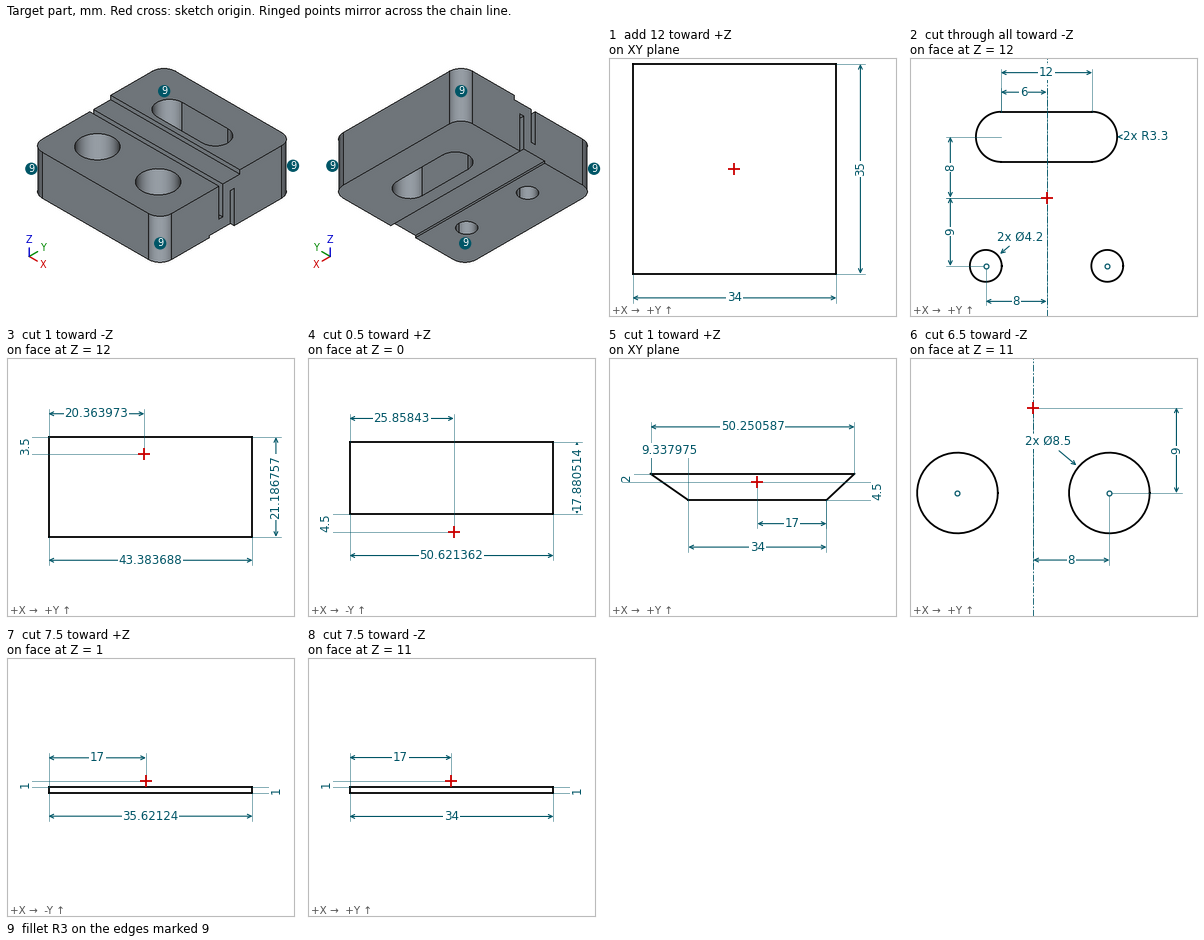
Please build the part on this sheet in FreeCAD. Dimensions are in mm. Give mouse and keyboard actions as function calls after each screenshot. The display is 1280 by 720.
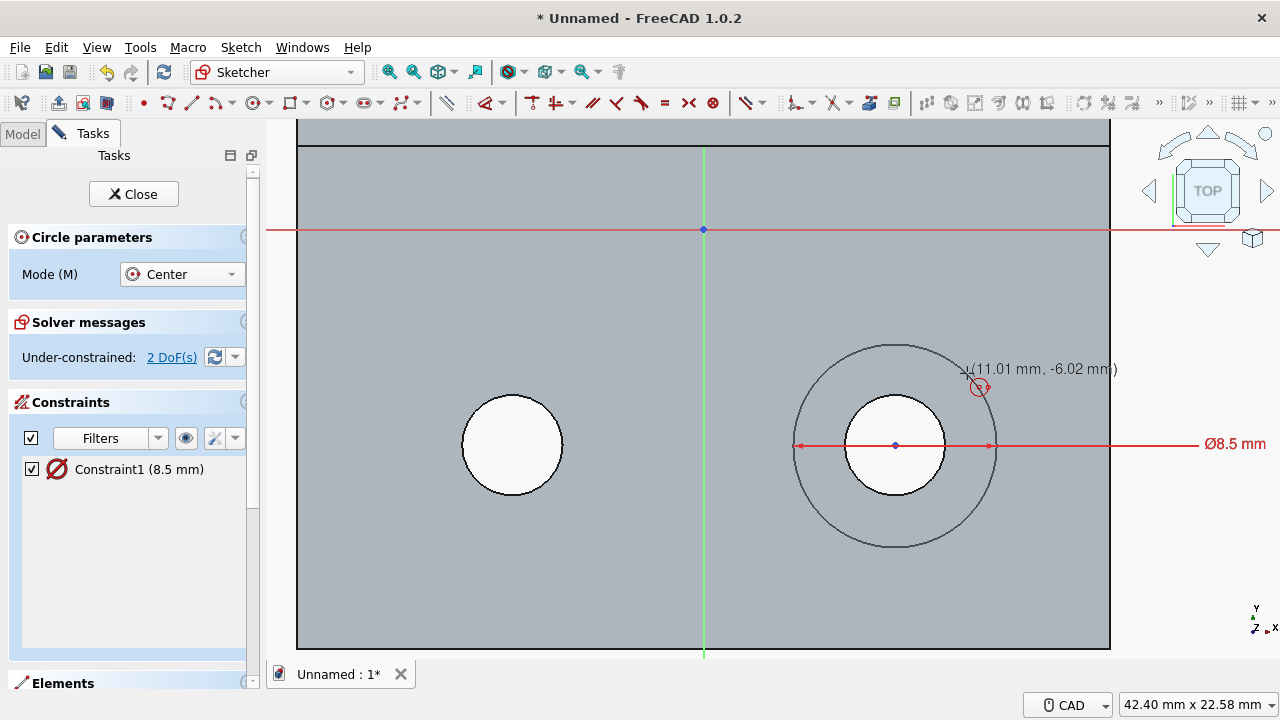
click(512, 445)
move(584, 373)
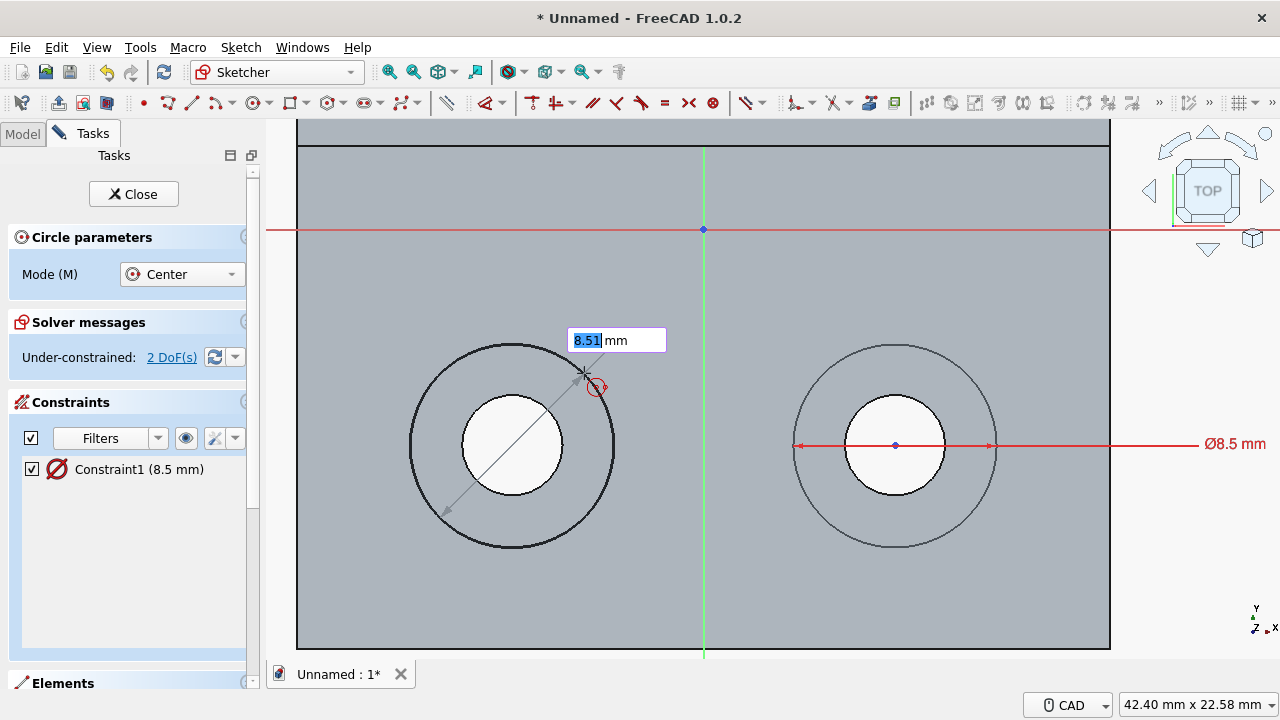
text(8.5)
key(Return)
key(Escape)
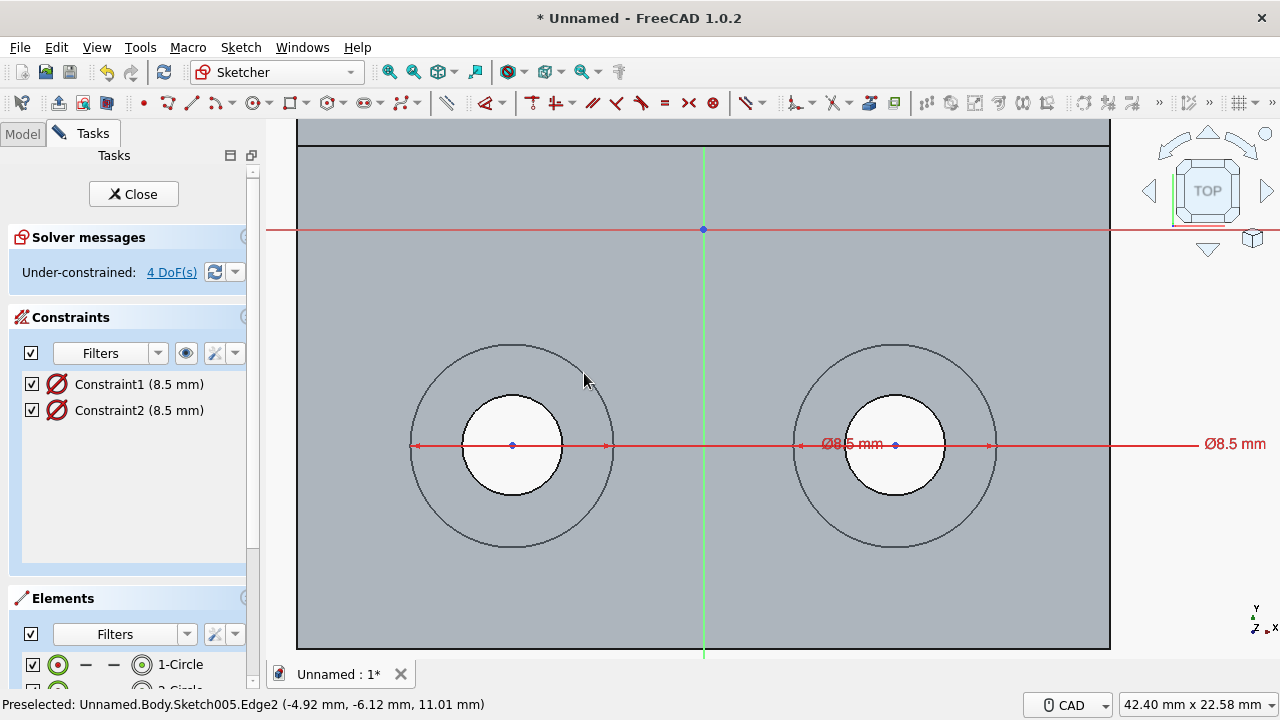
click(895, 446)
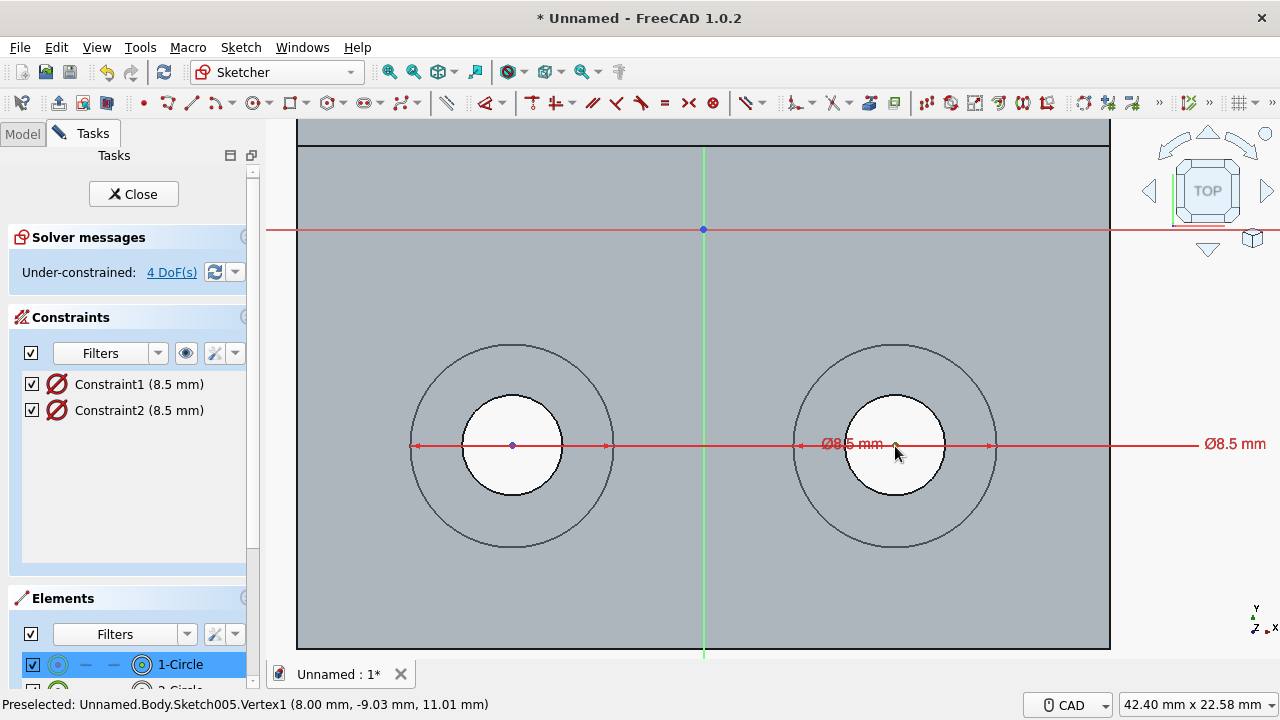
click(512, 446)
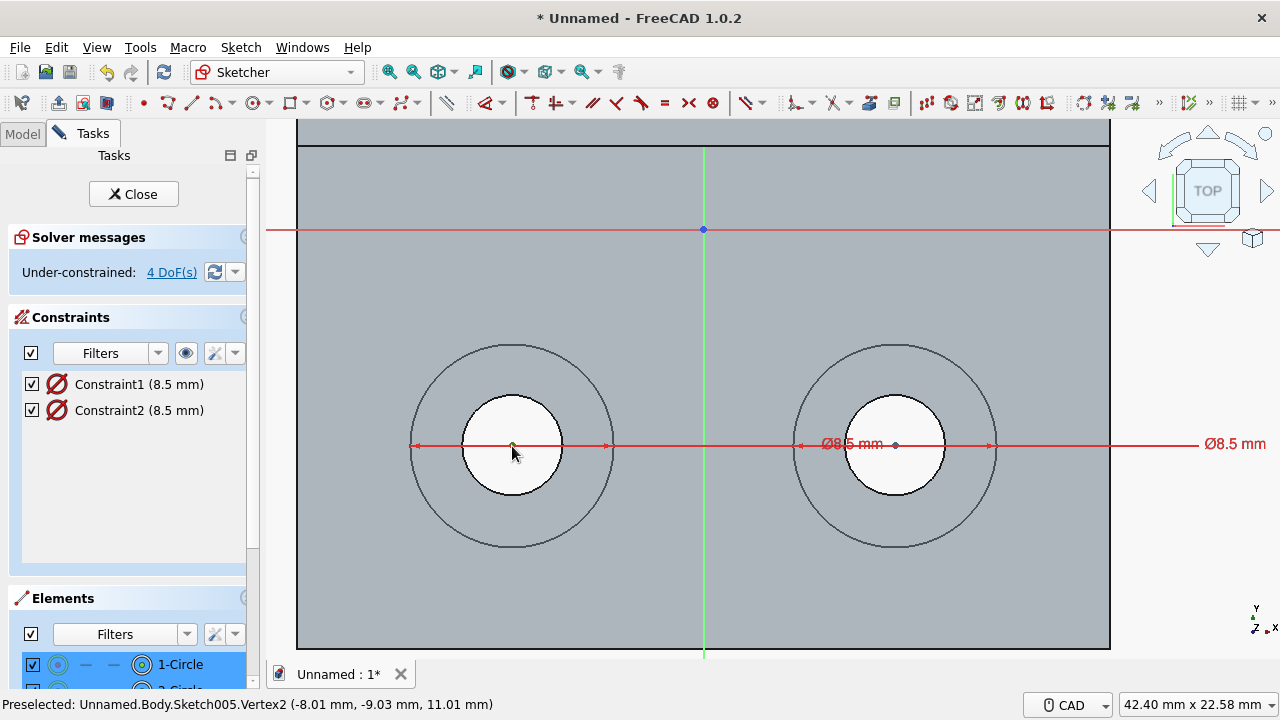
click(704, 596)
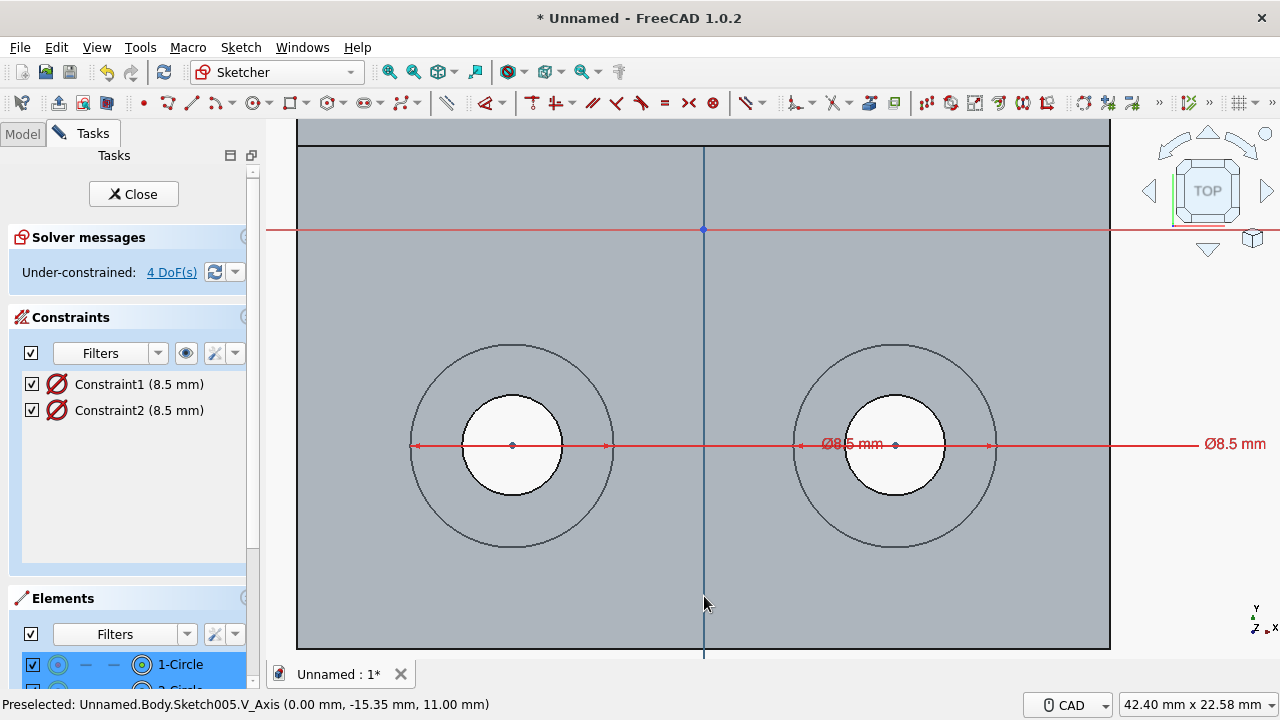
key(s)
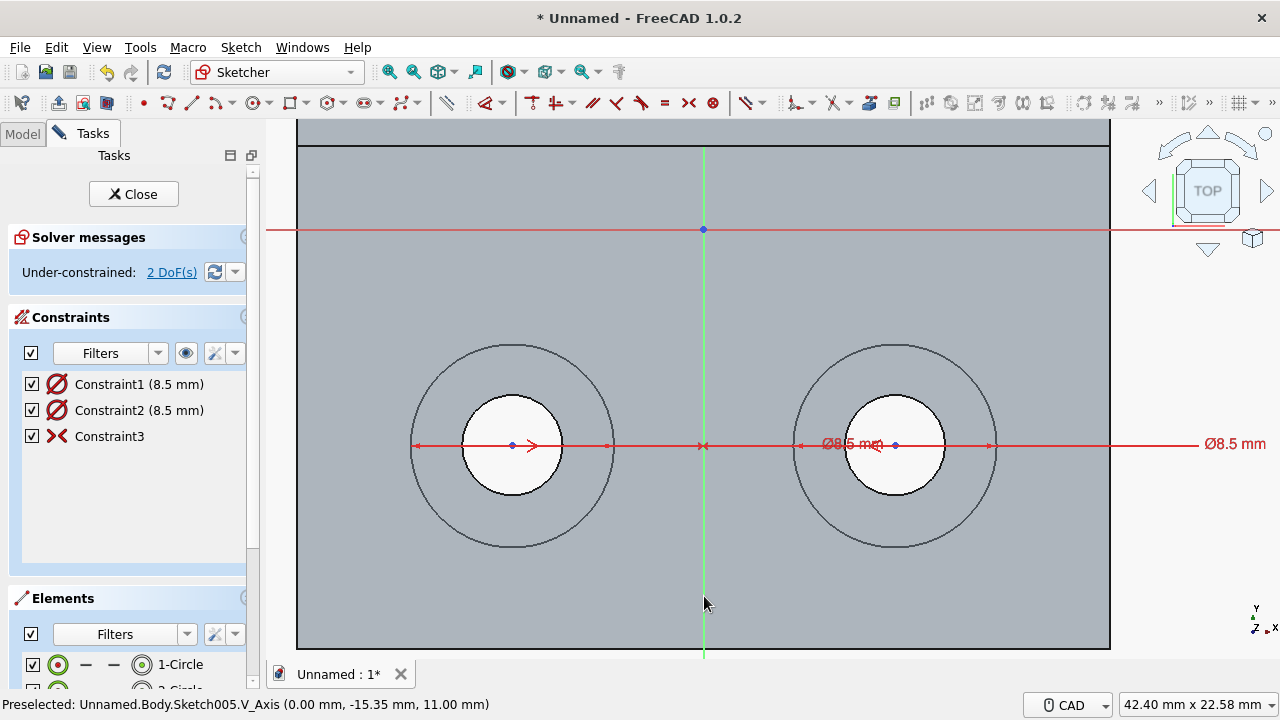
key(d)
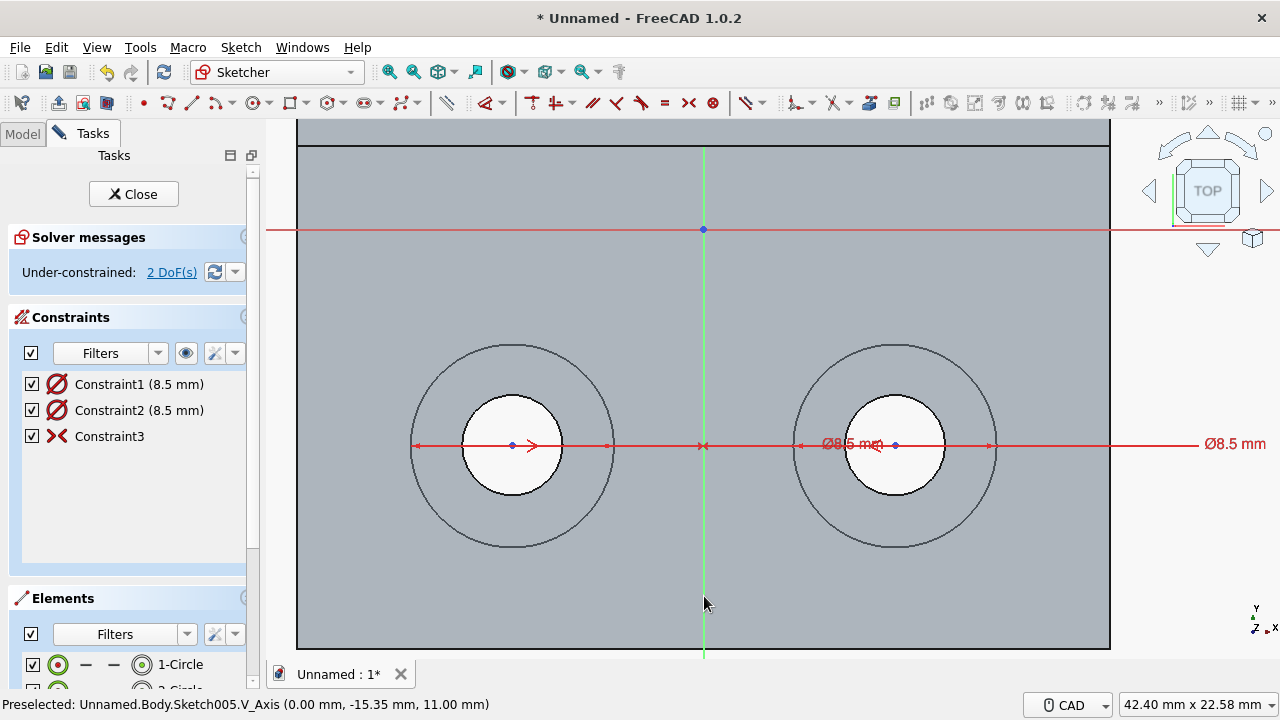
click(895, 446)
click(799, 196)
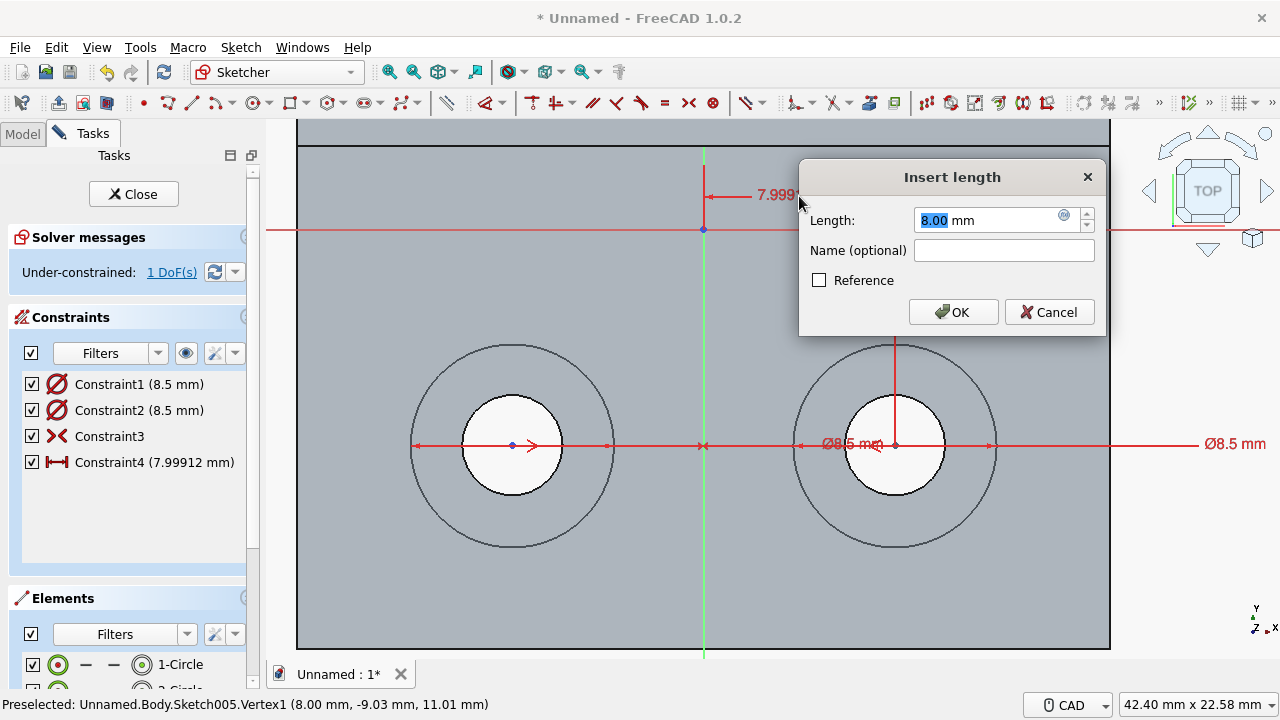
text(8)
key(Return)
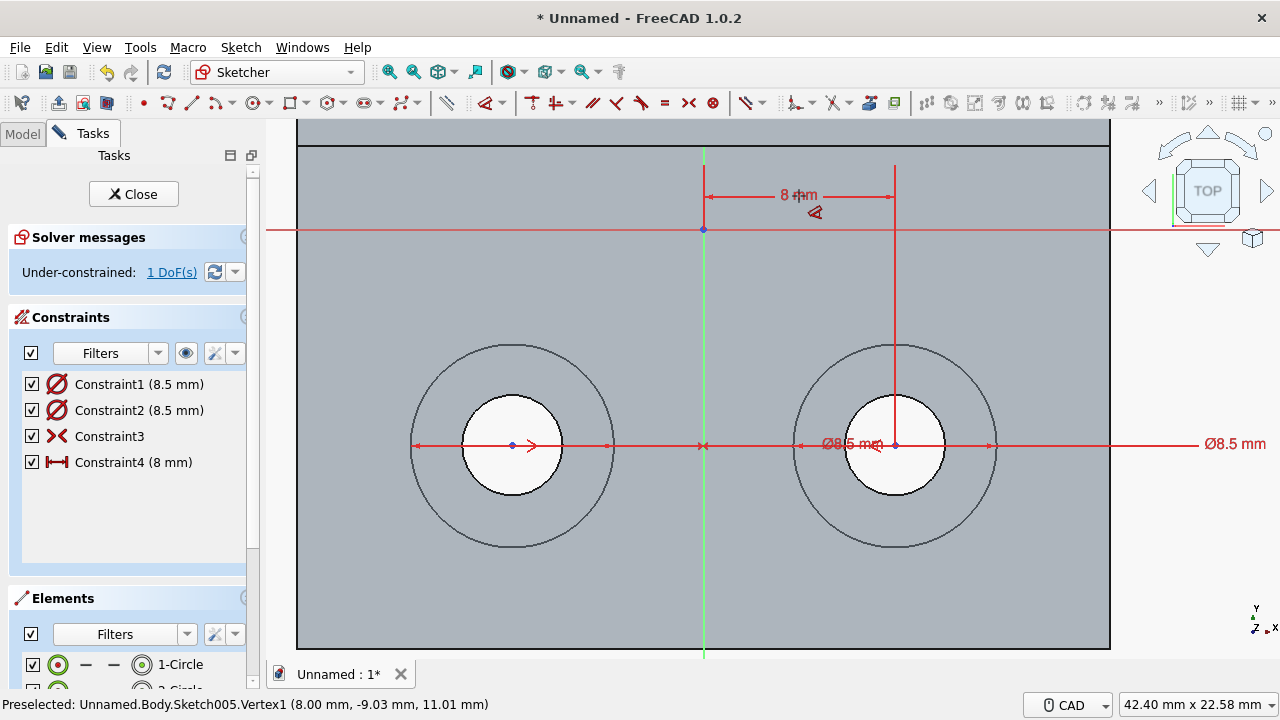
click(895, 446)
click(929, 288)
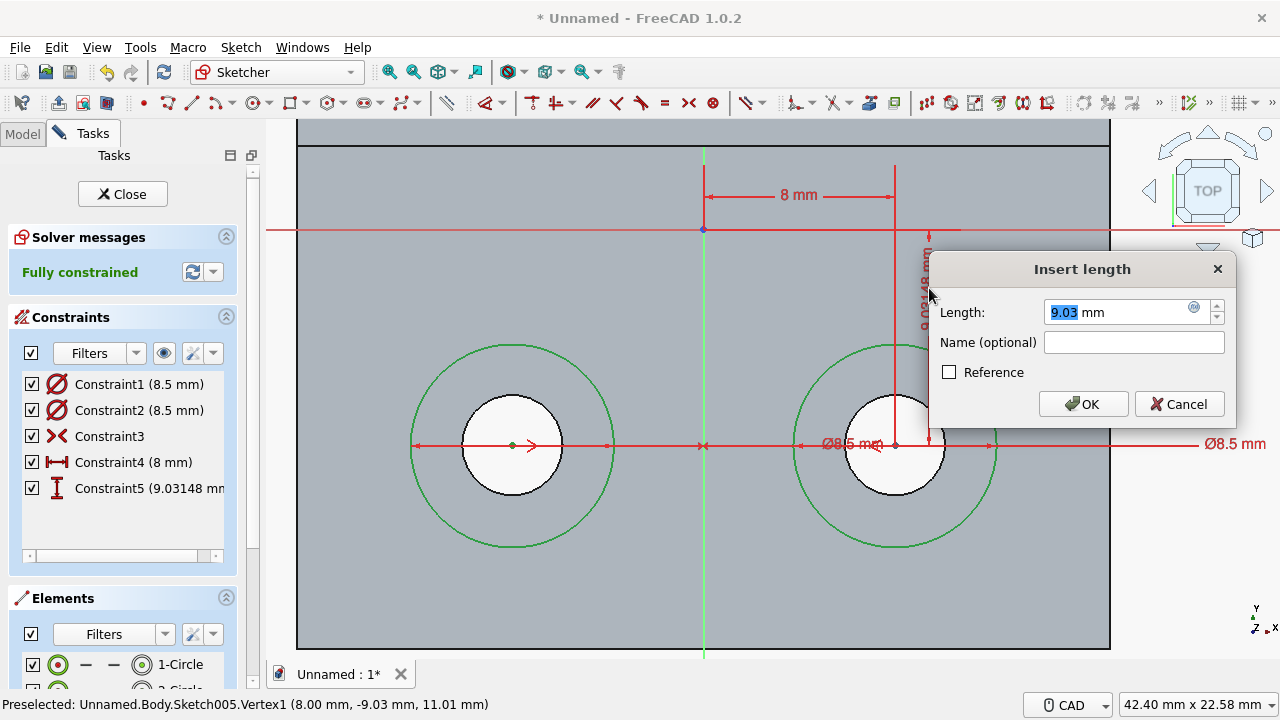
text(9)
key(Return)
key(Escape)